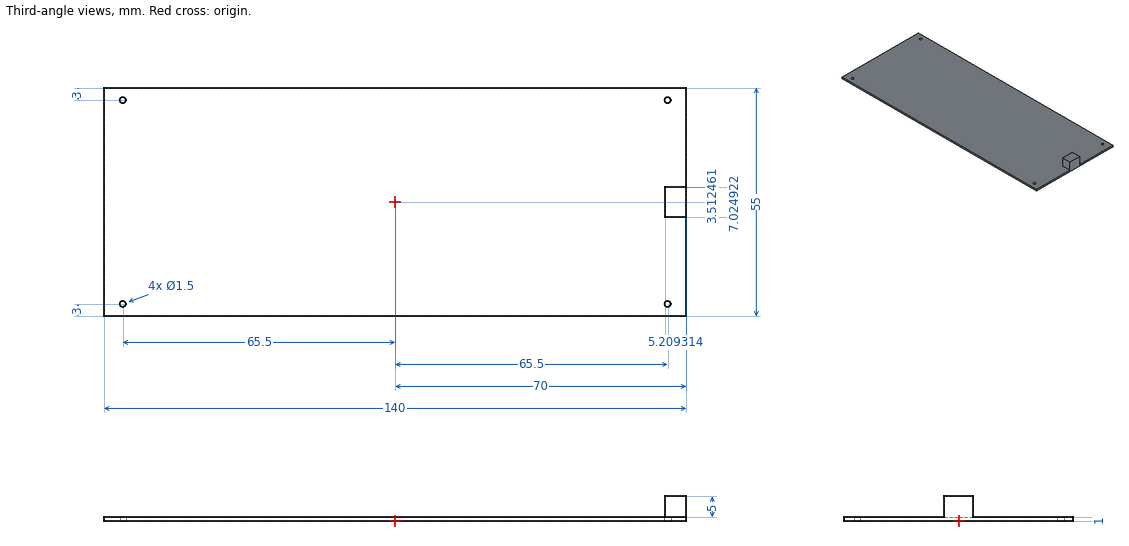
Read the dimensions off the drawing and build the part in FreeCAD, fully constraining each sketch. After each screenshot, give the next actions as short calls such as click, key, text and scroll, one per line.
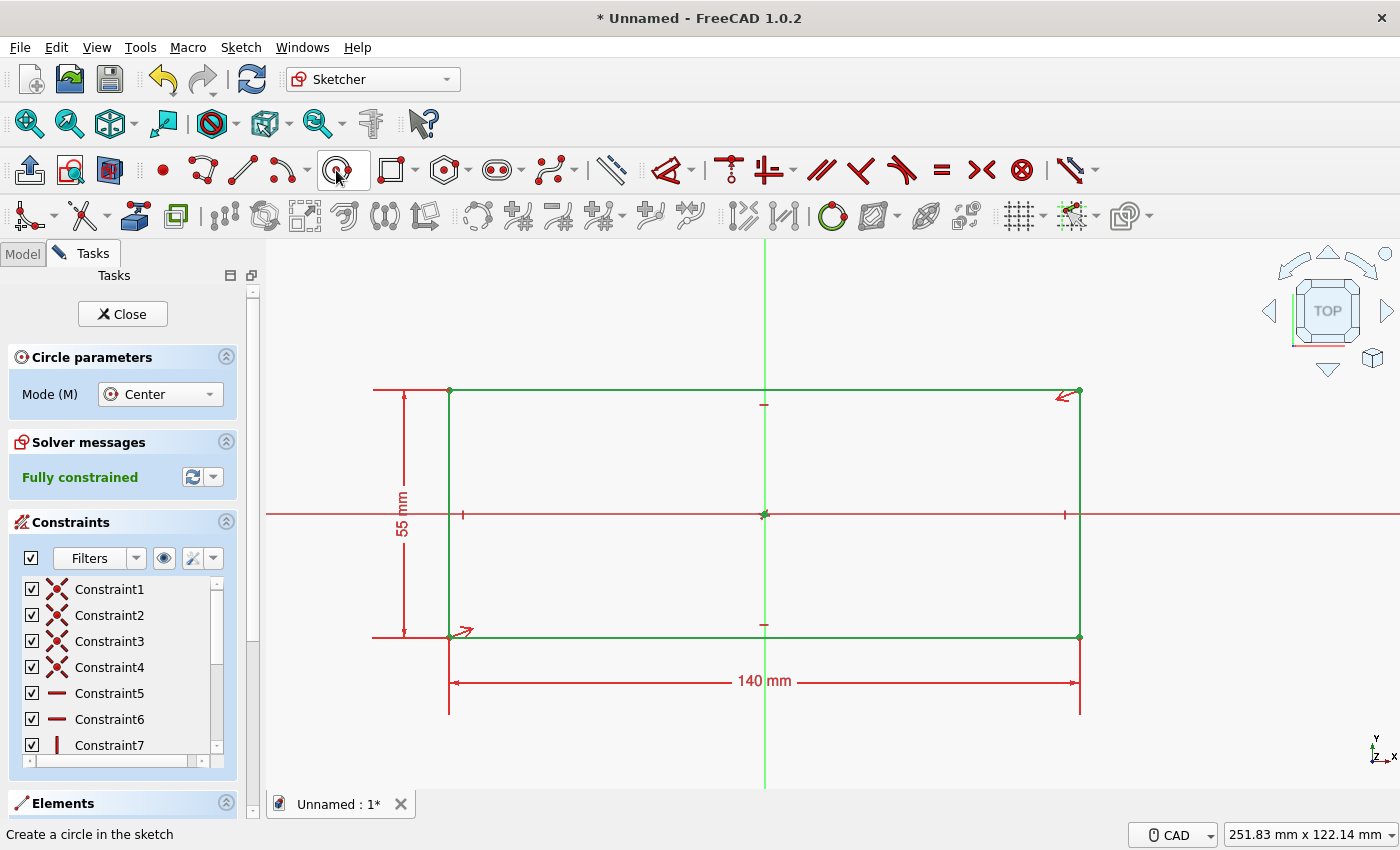
scroll(470, 624, up, 10)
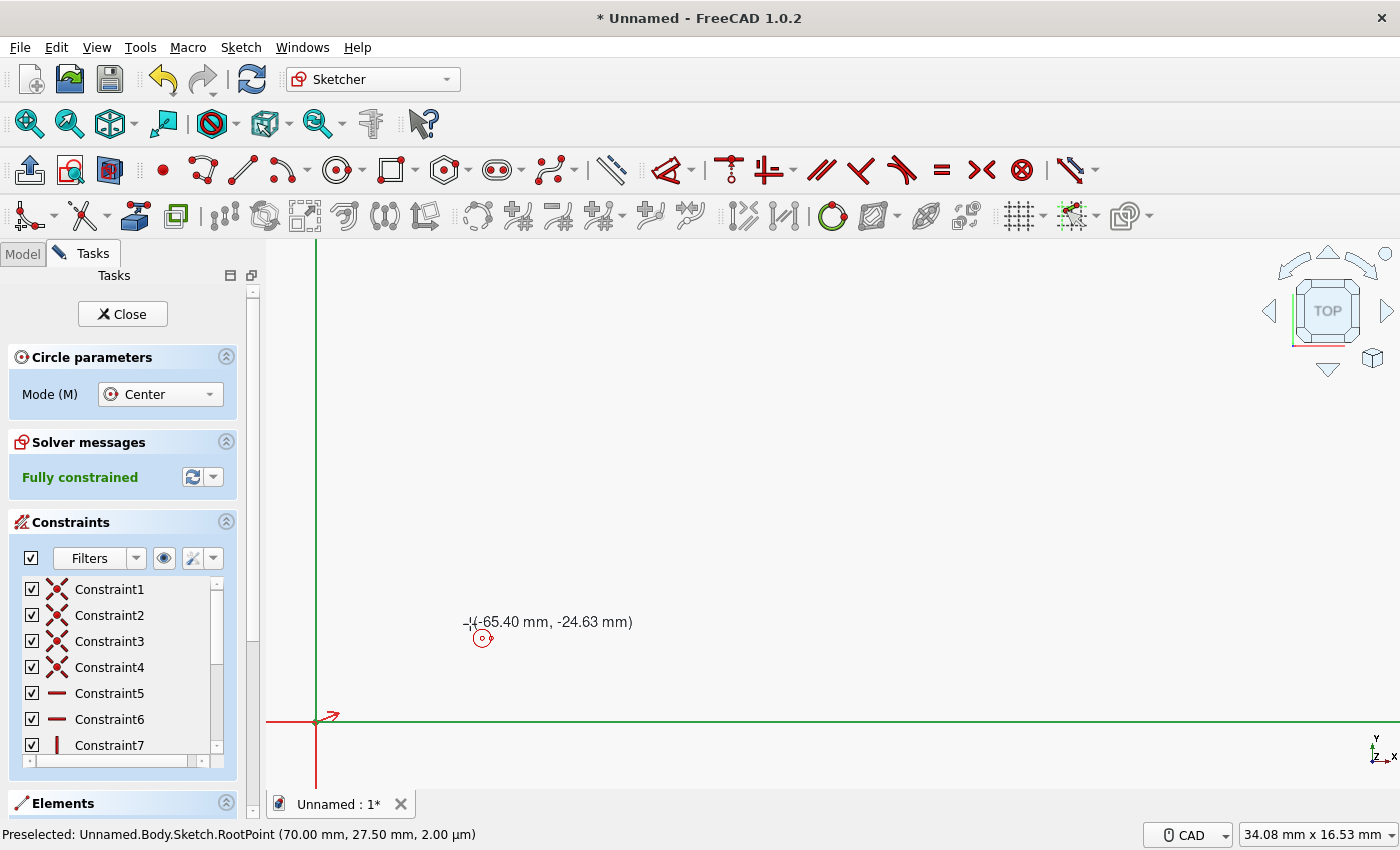
scroll(470, 625, down, 10)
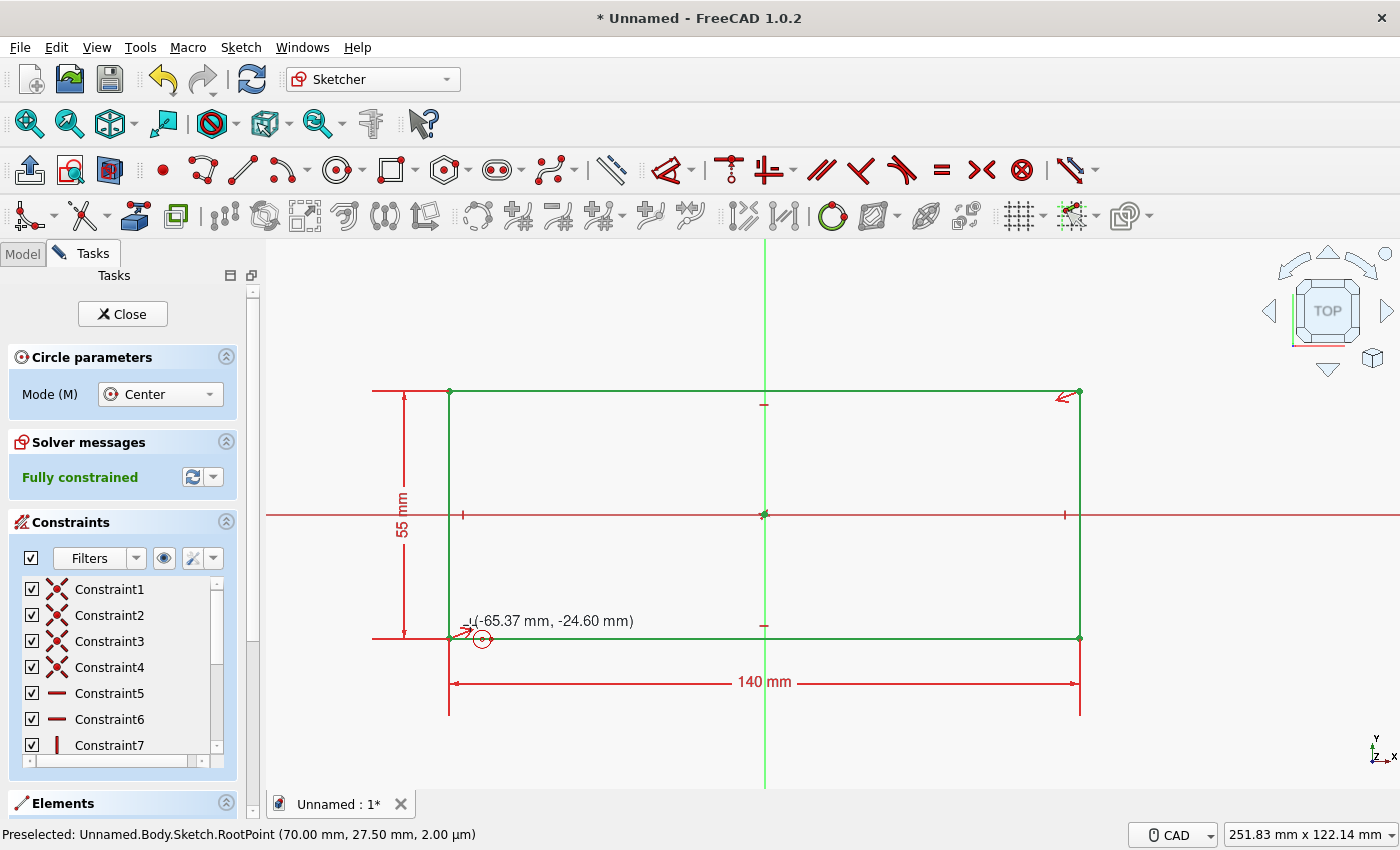
click(470, 625)
move(472, 623)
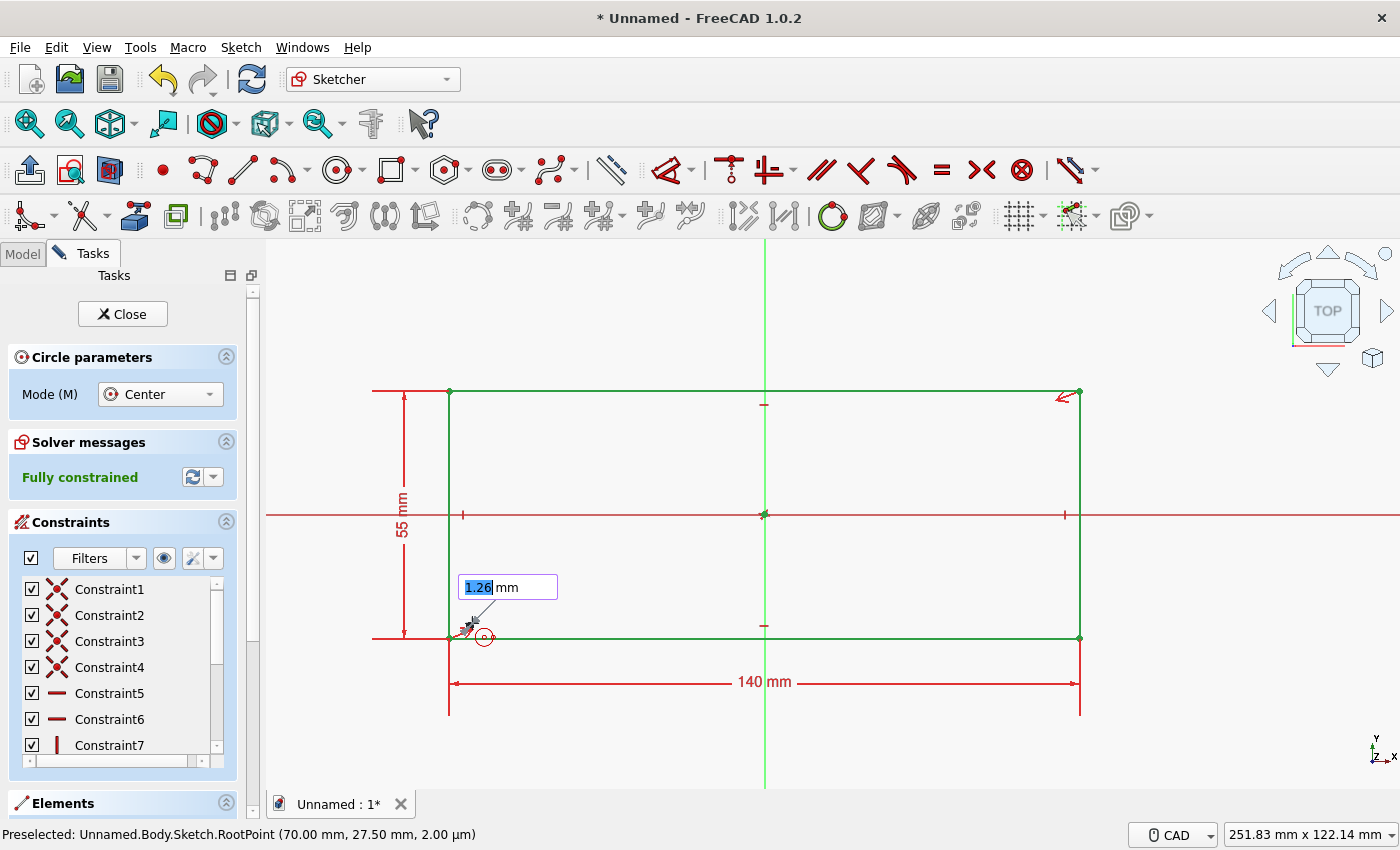
text(1.5)
key(Return)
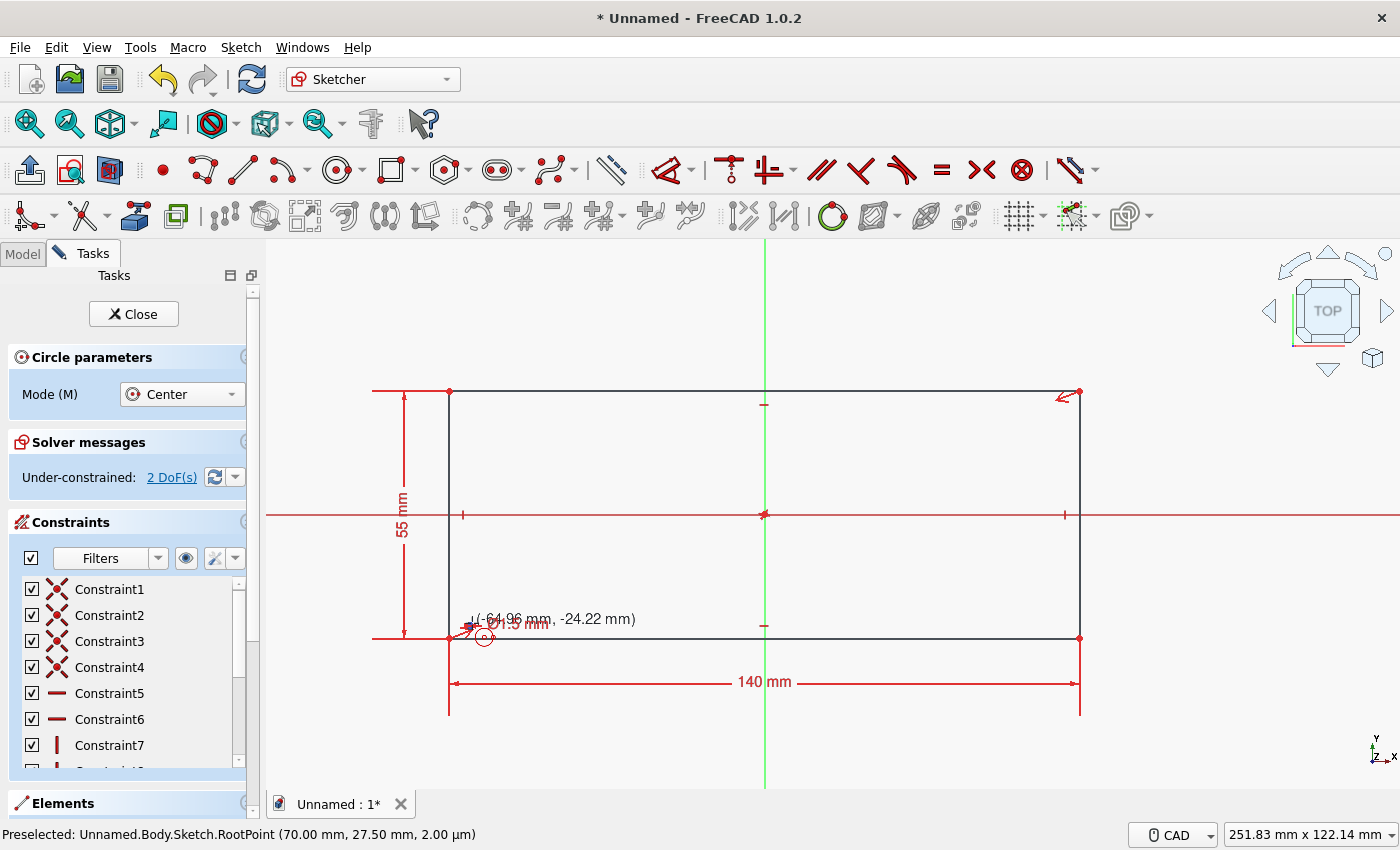
scroll(1059, 625, up, 10)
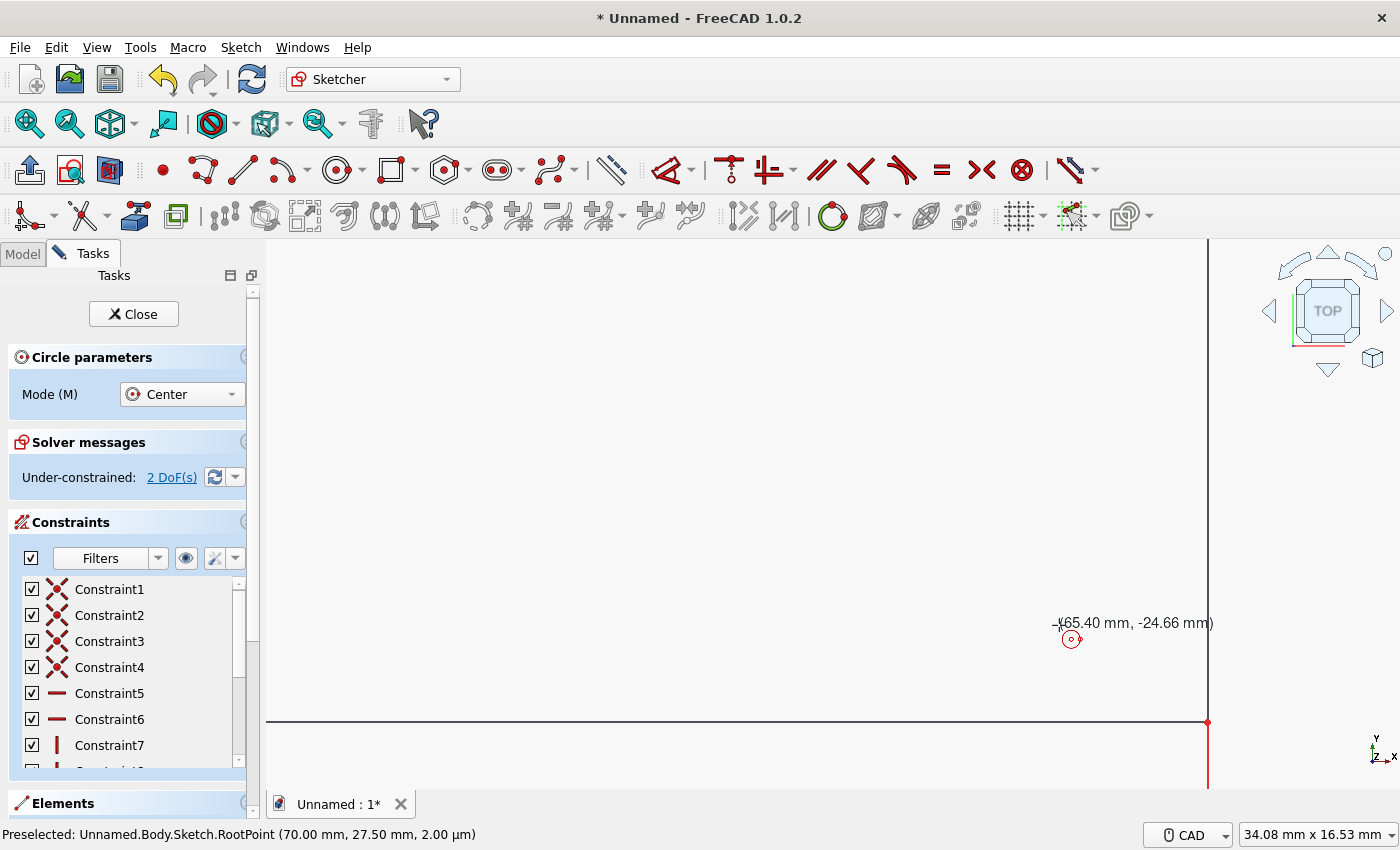
scroll(1060, 625, down, 10)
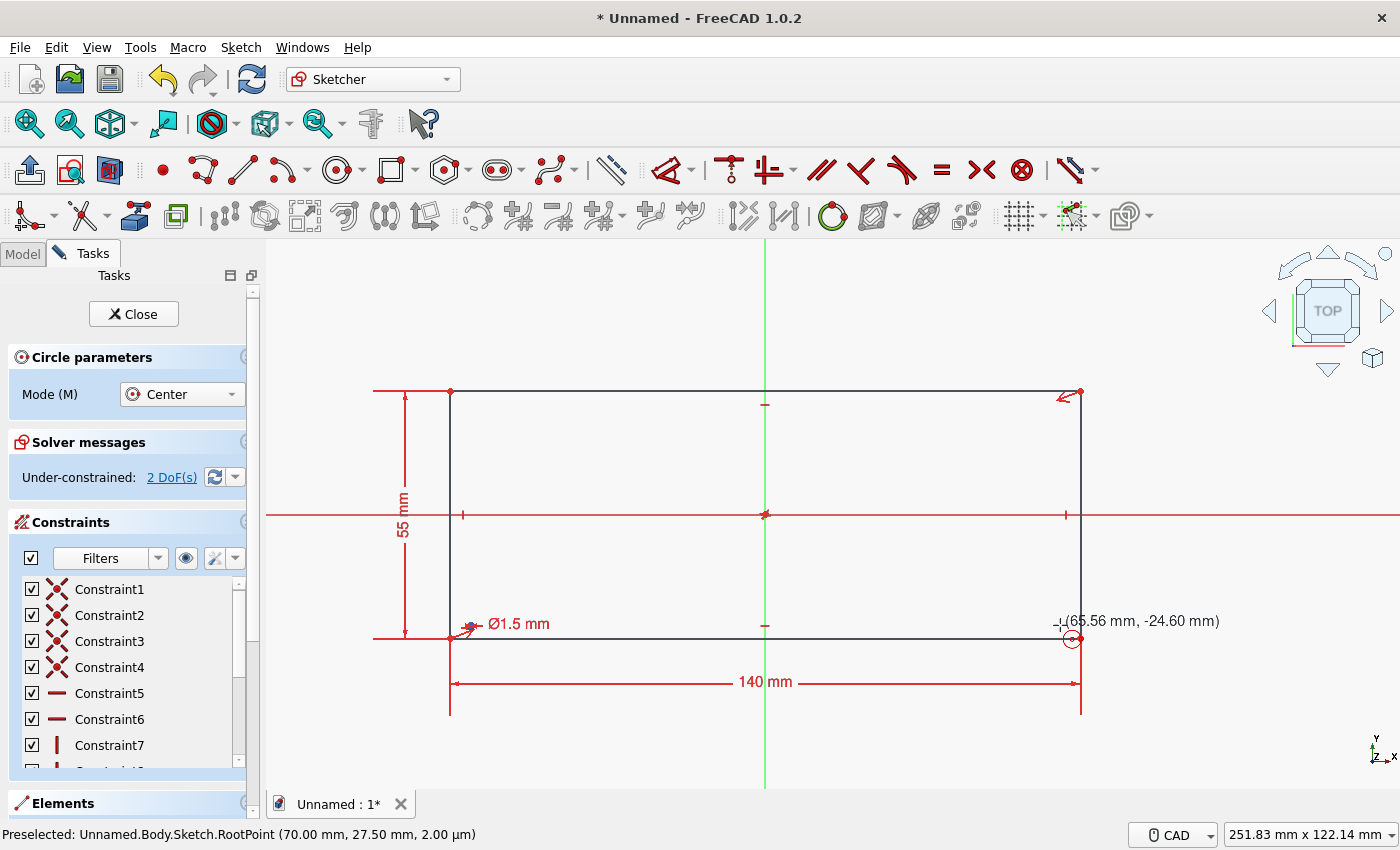
click(1060, 625)
move(1063, 623)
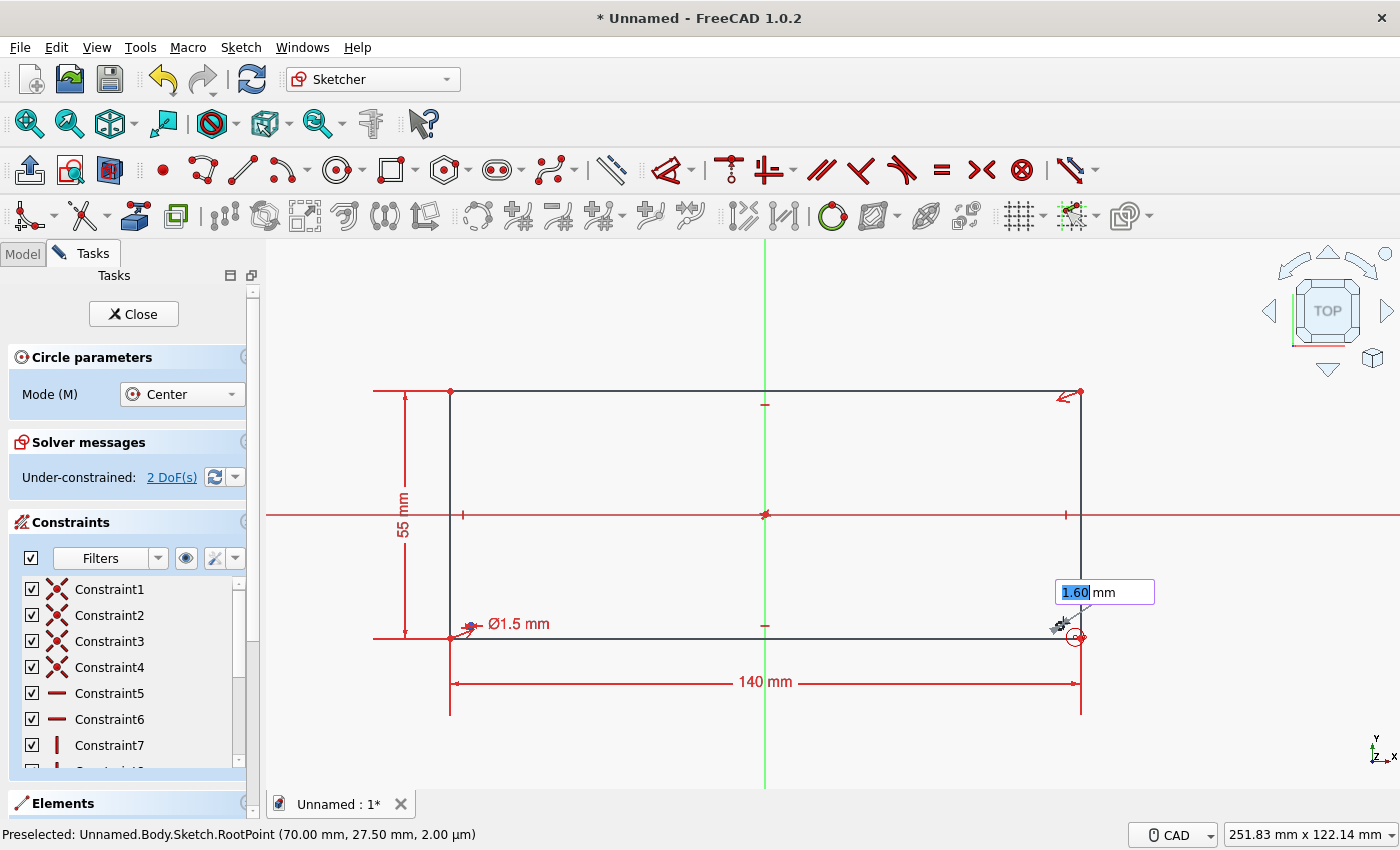
text(1.5)
key(Return)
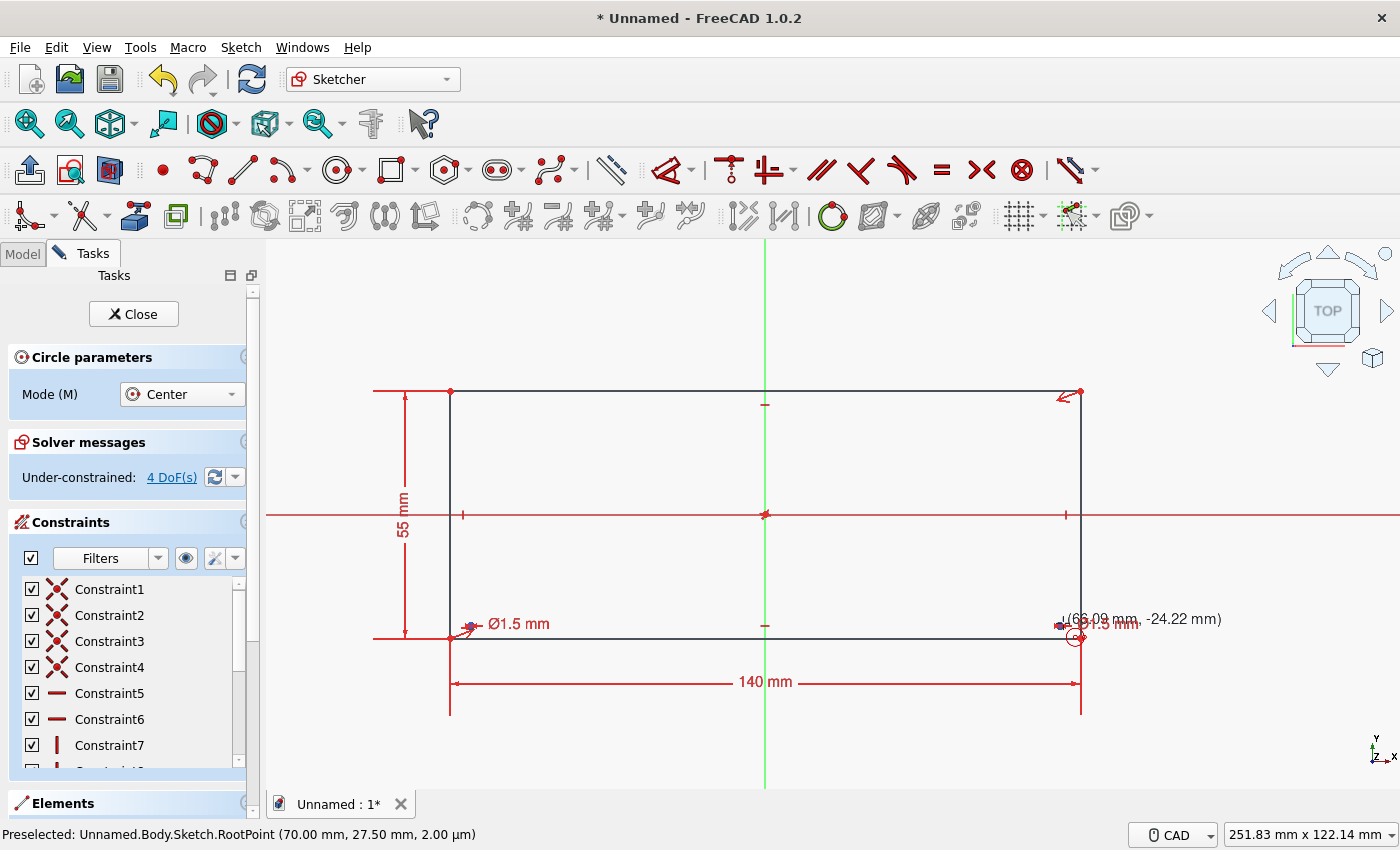
scroll(470, 405, up, 10)